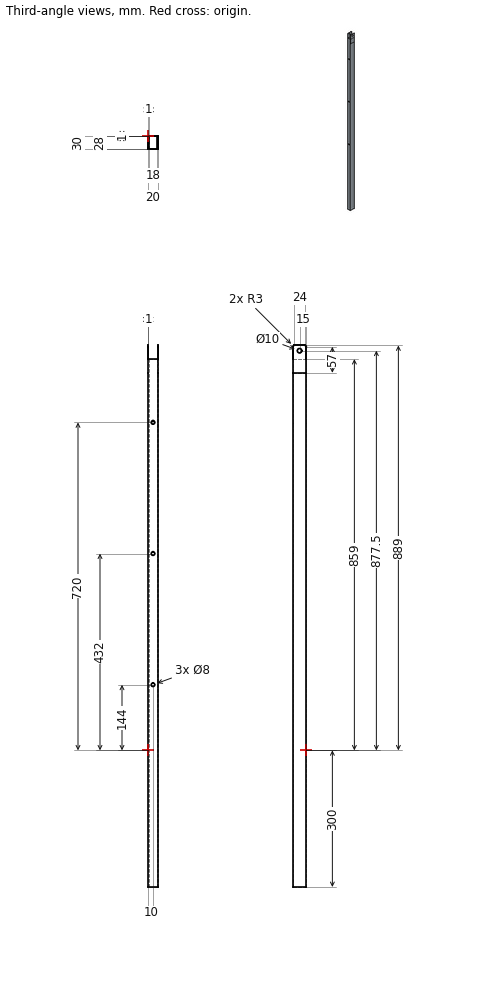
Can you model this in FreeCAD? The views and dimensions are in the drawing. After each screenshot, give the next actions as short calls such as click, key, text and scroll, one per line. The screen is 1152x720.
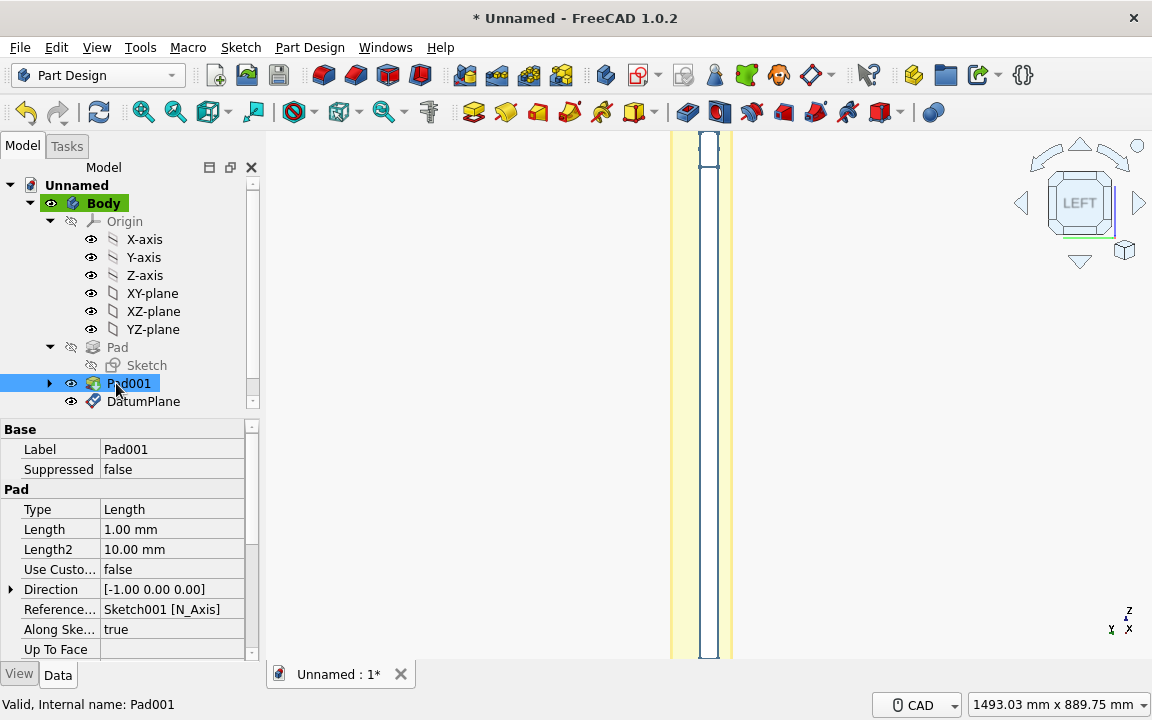
click(466, 76)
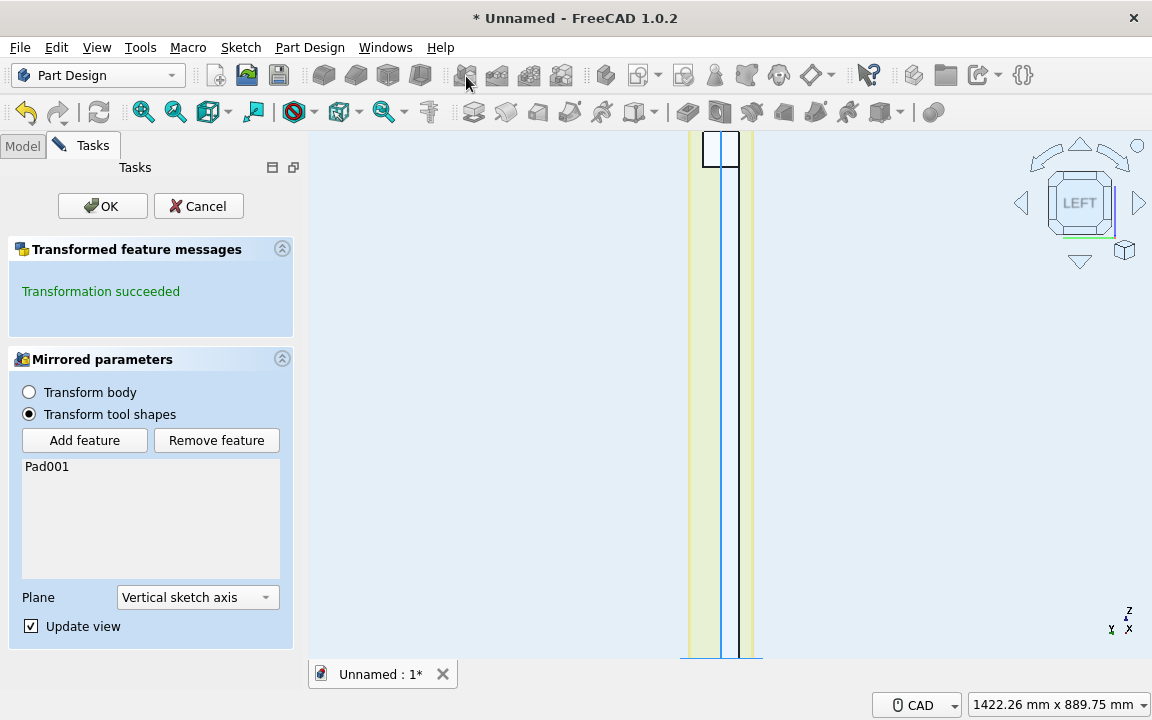
click(198, 598)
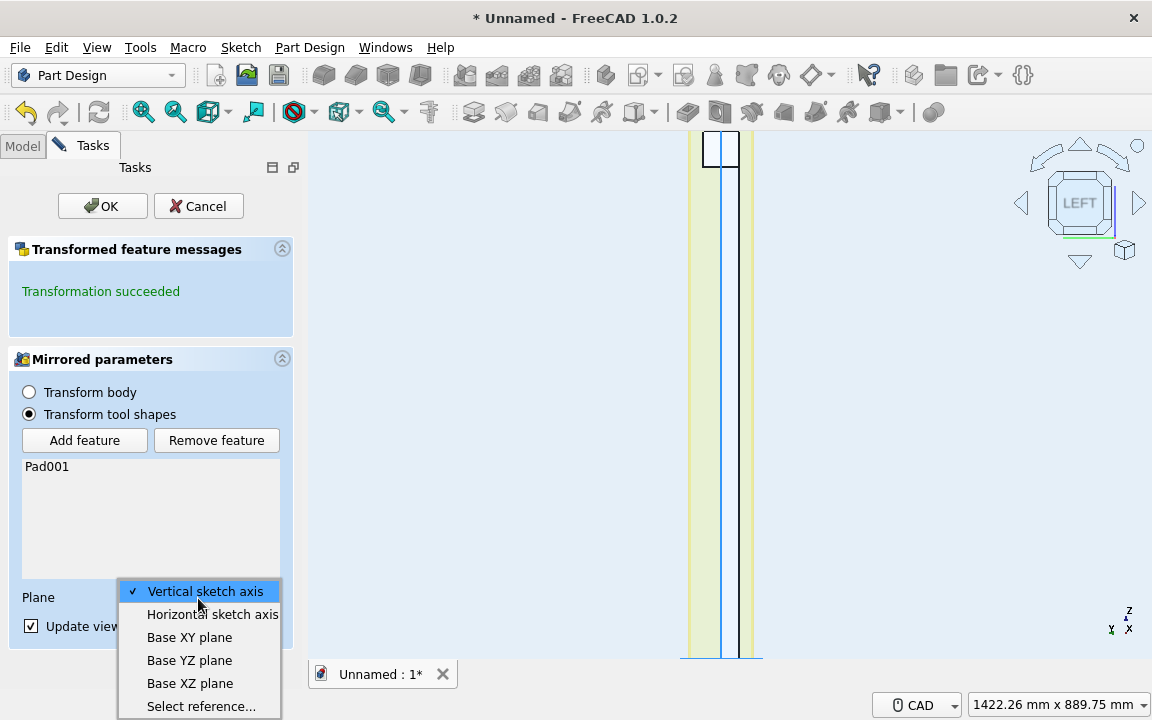
click(198, 706)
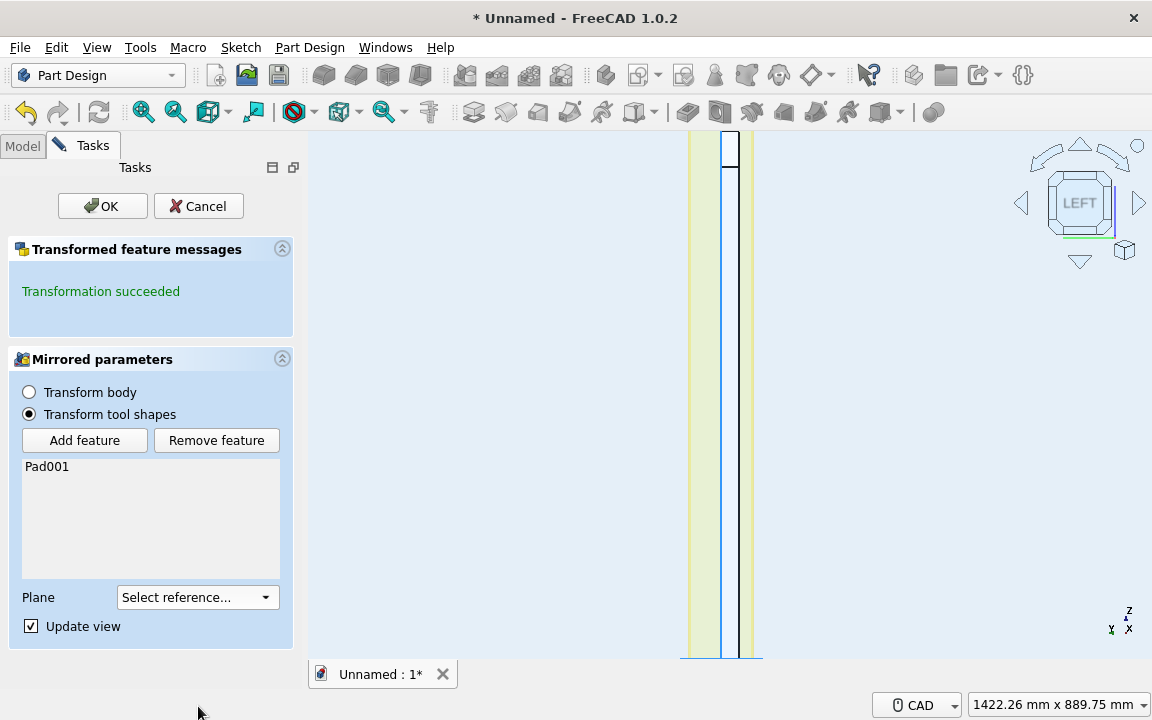
click(23, 145)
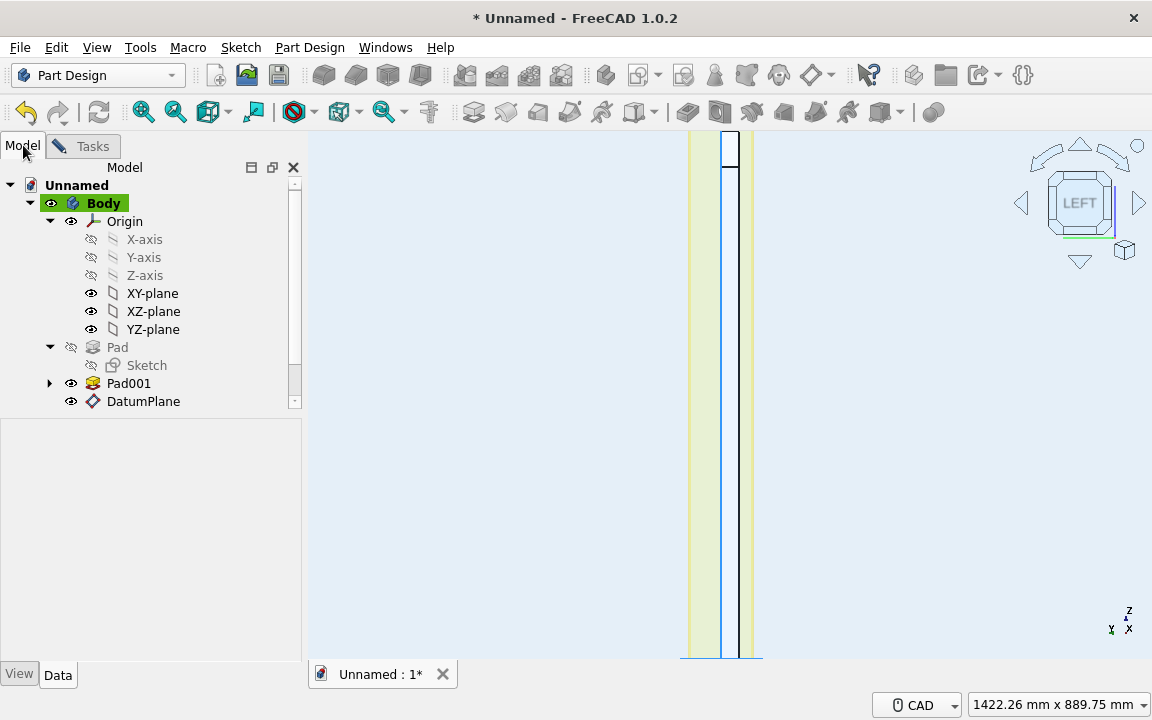
click(116, 401)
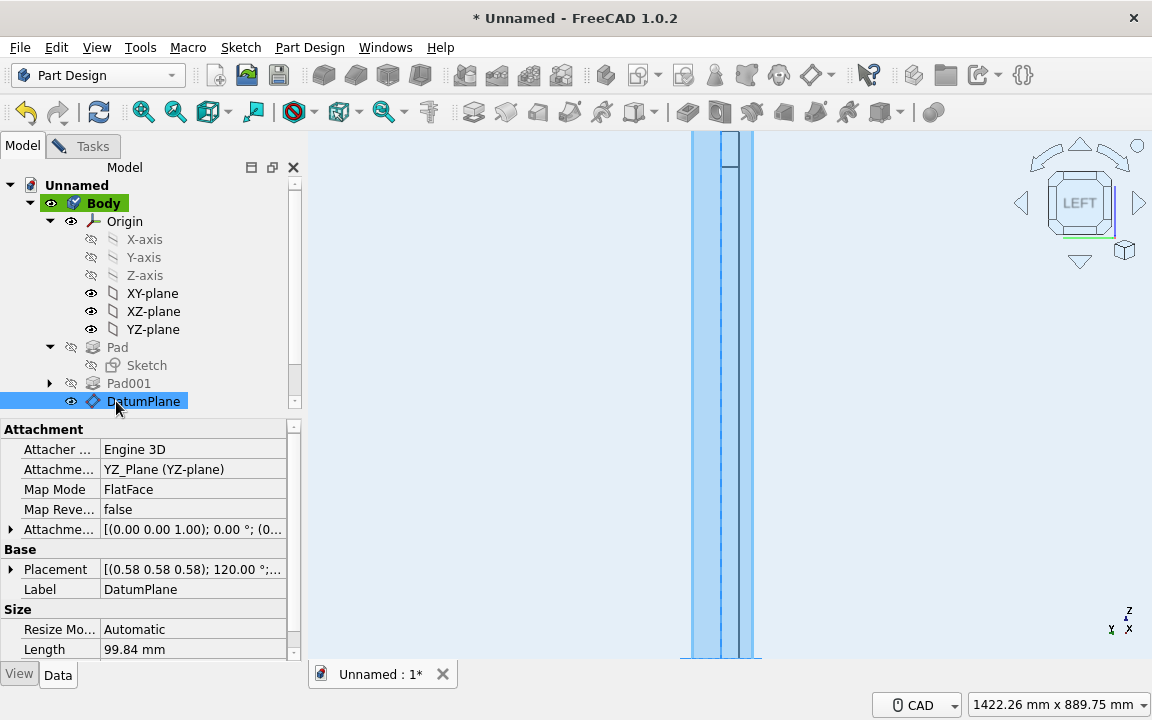
click(84, 145)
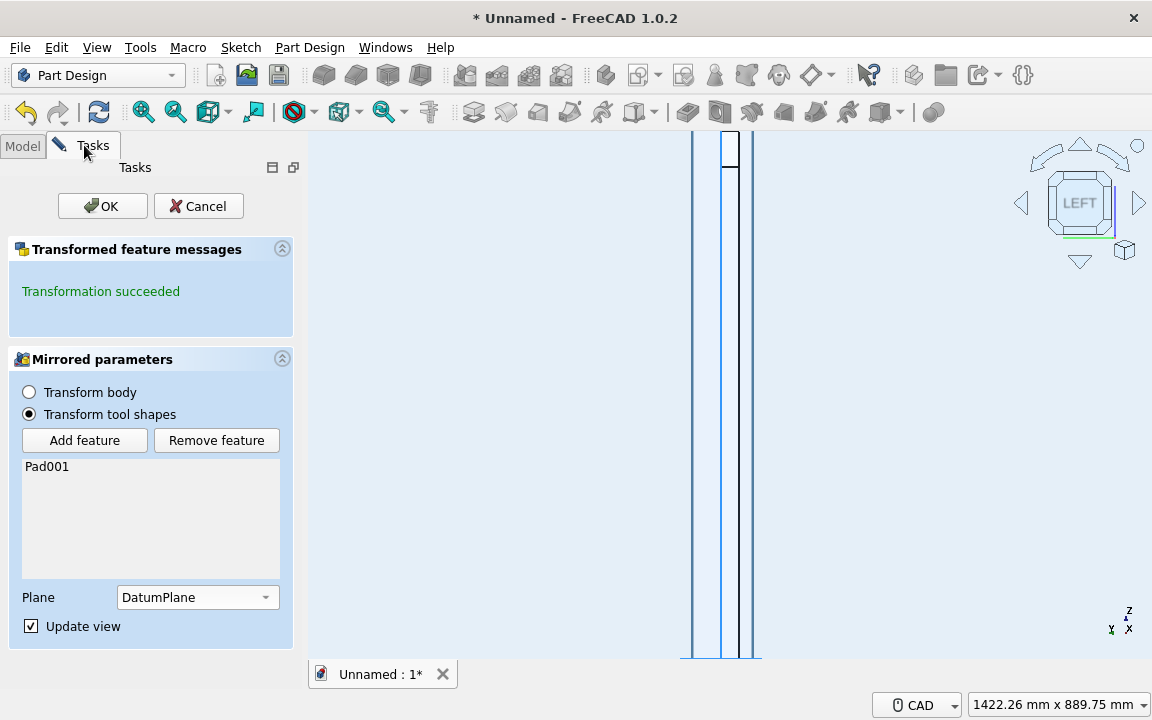
click(103, 206)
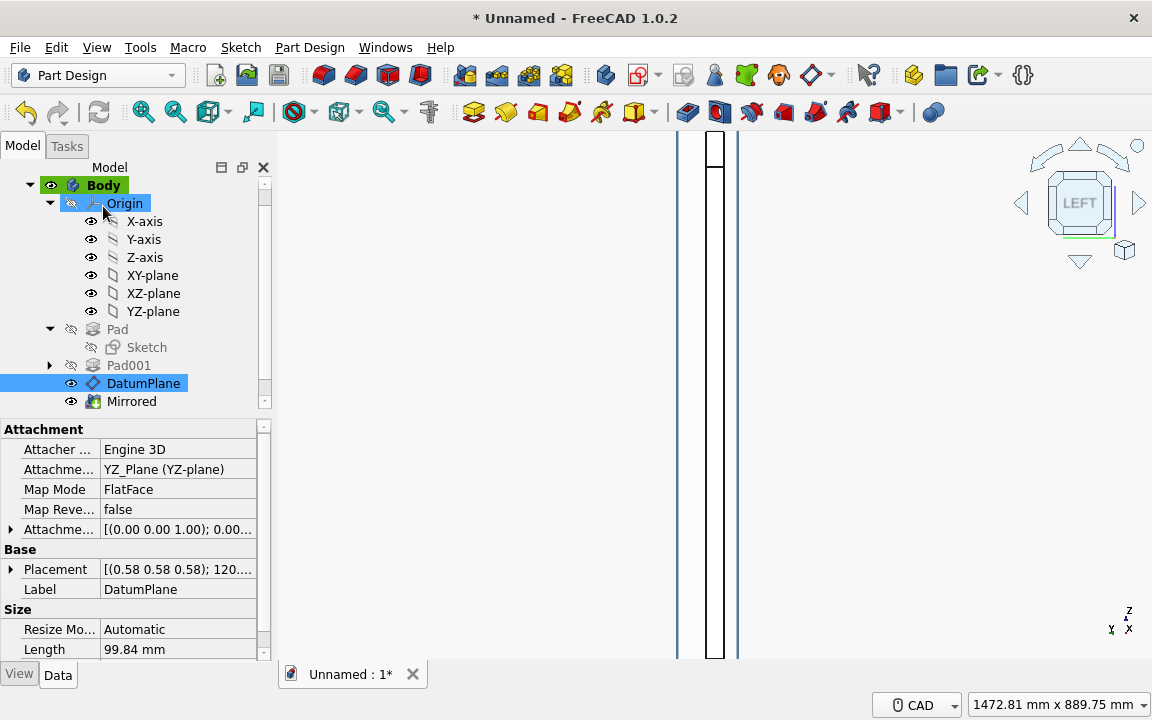
click(116, 383)
key(space)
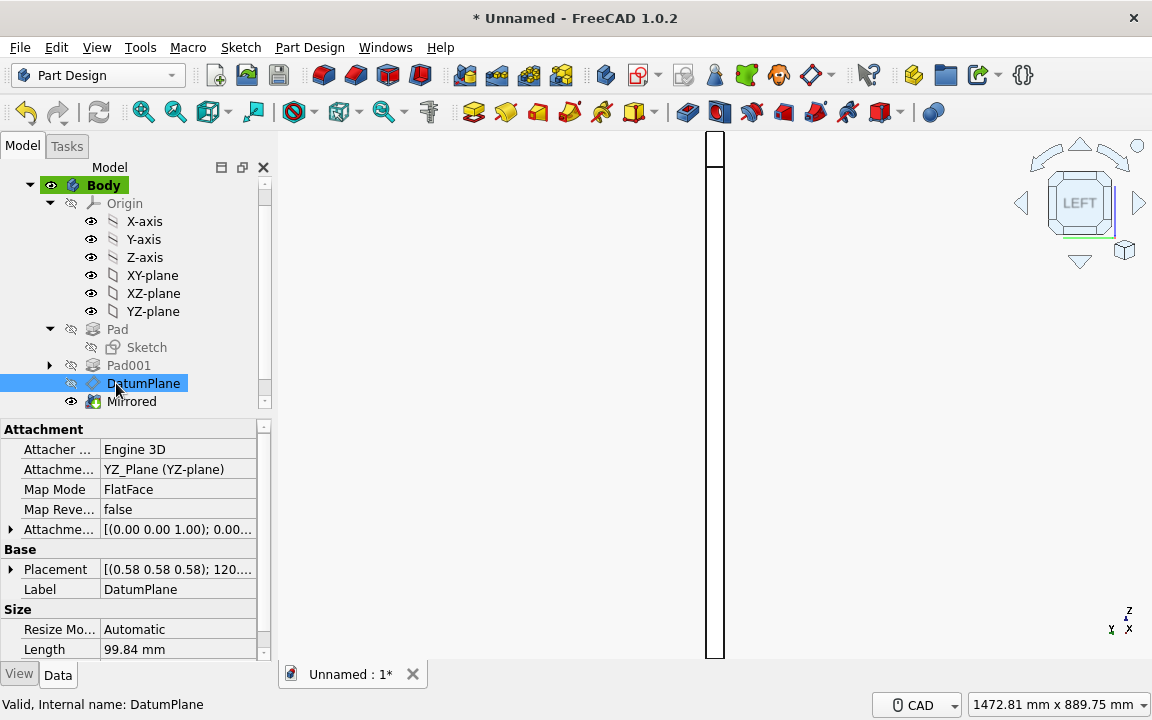
key(v)
key(f)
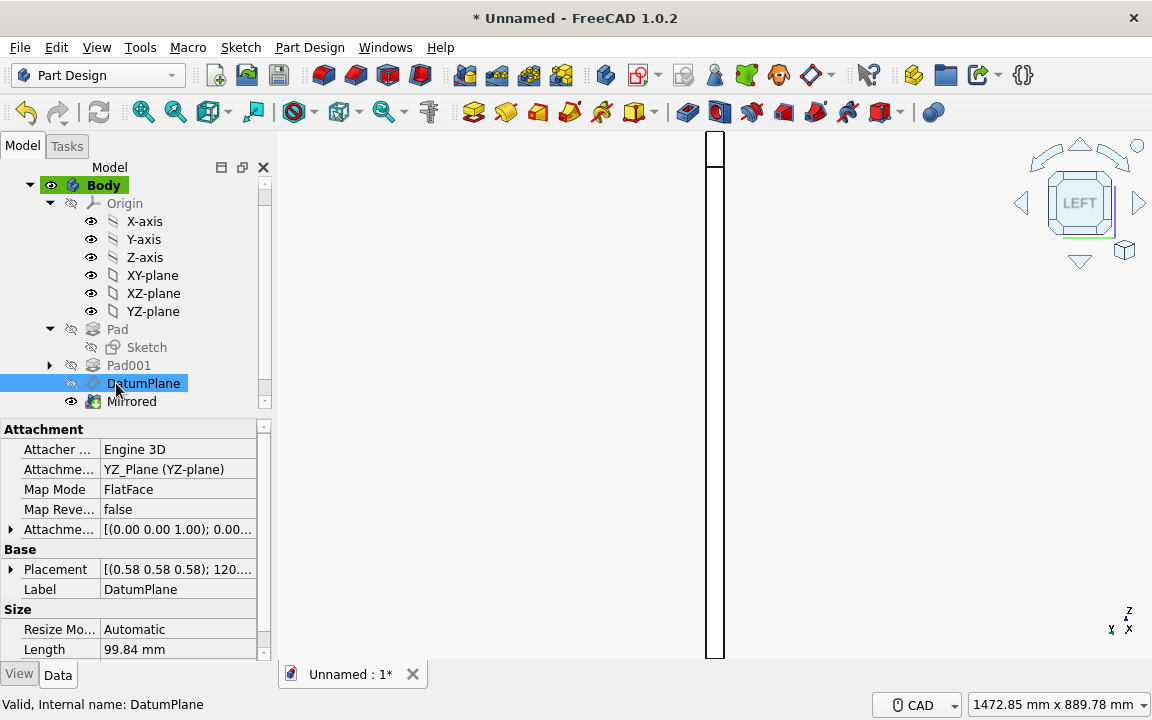
key(0)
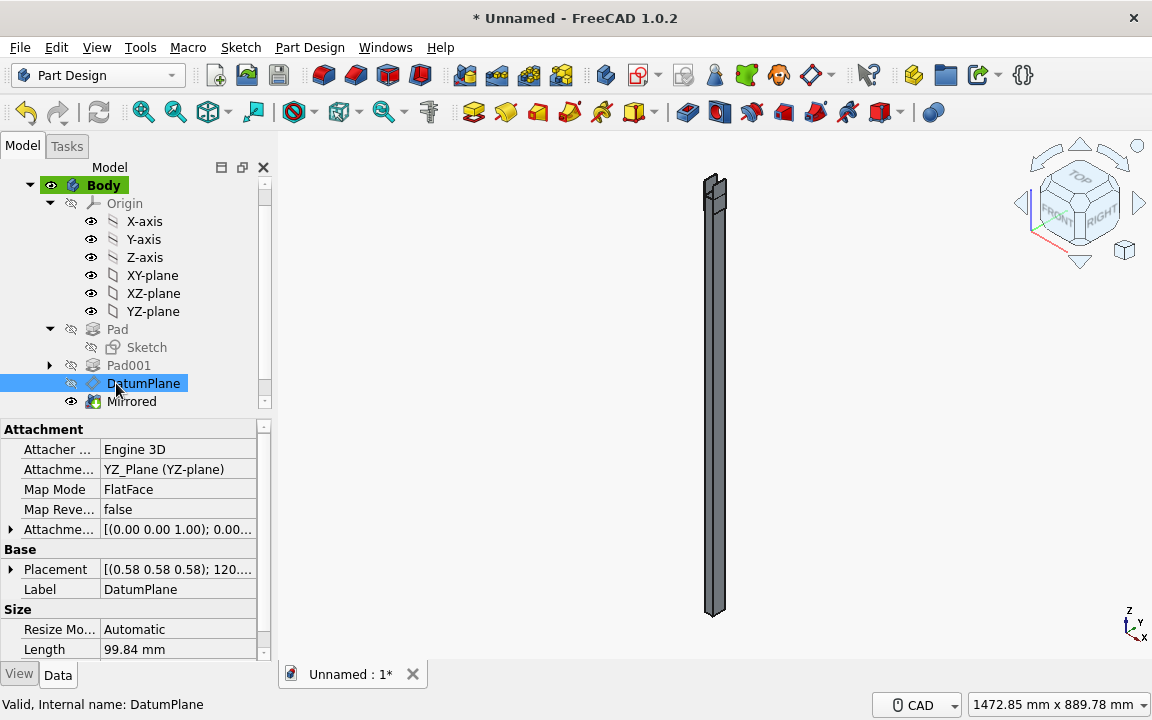
key(3)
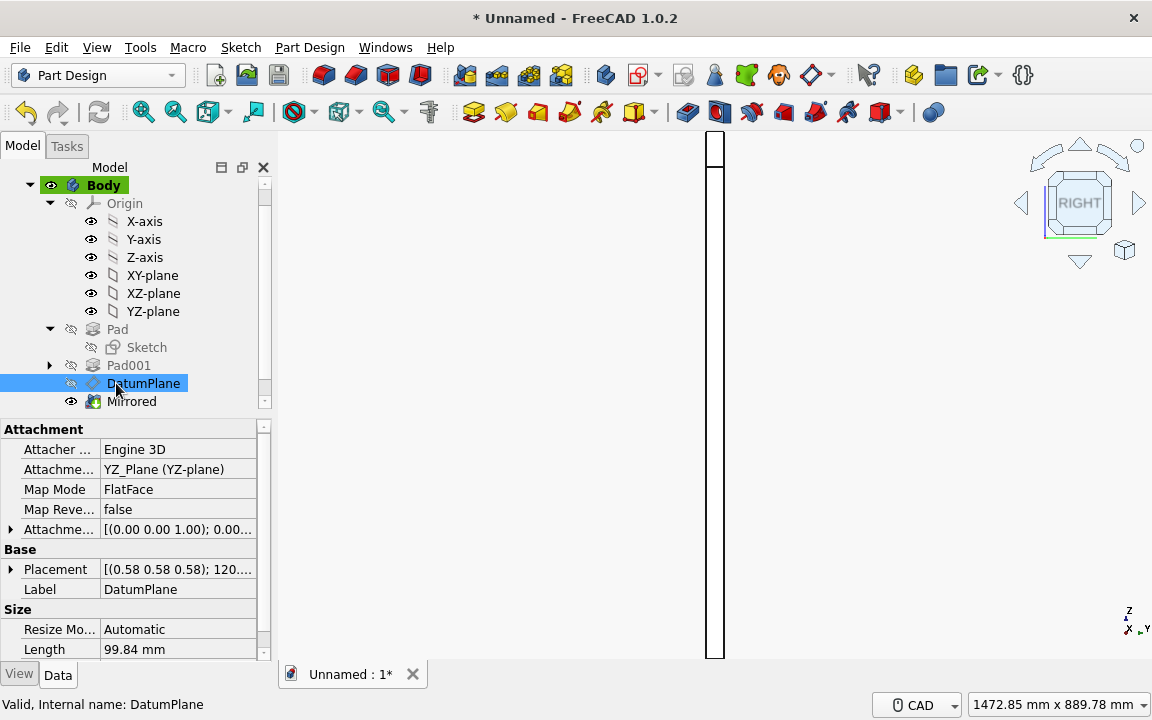
click(144, 112)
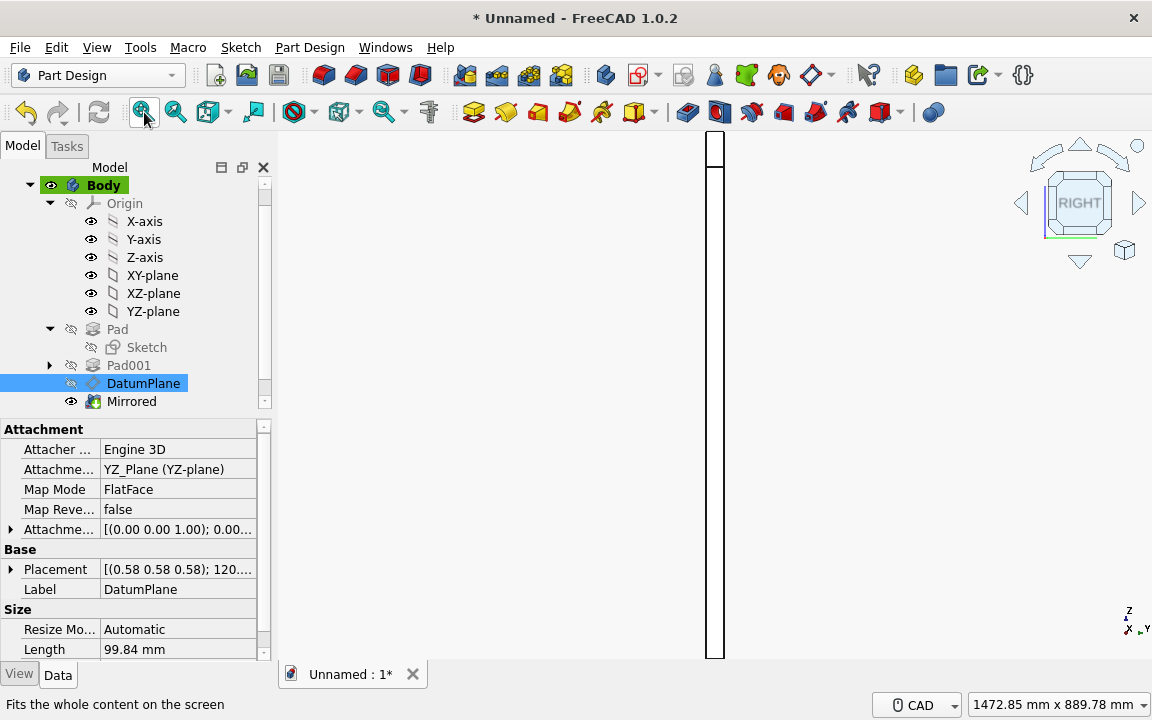
key(2)